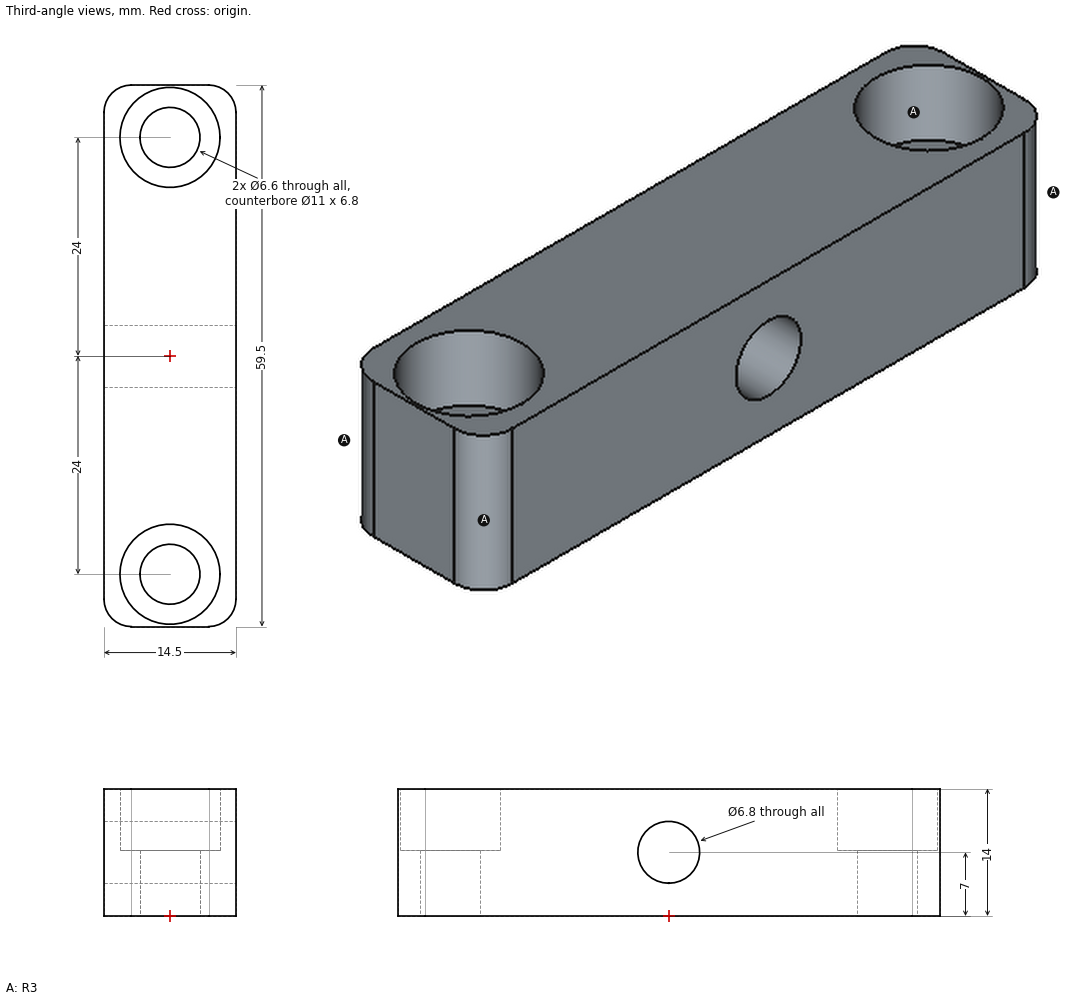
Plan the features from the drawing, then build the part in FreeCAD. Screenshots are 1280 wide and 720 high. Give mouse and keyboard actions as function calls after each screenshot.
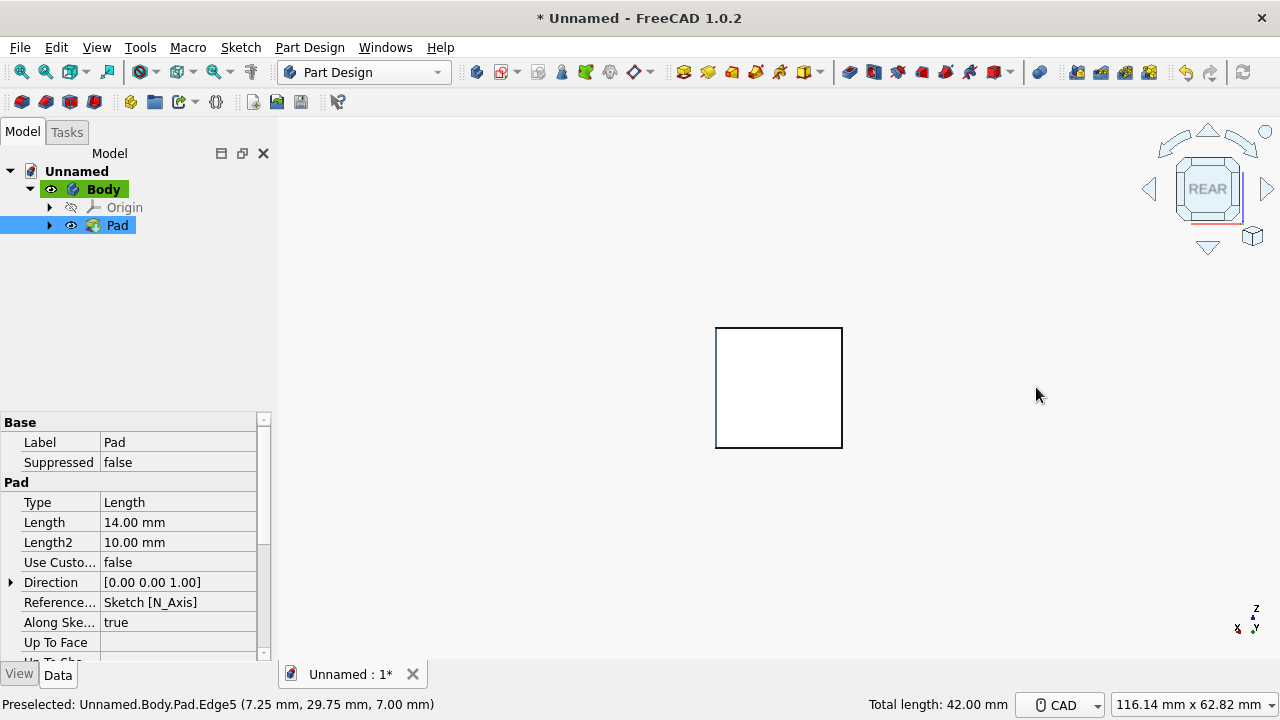
key(v)
key(f)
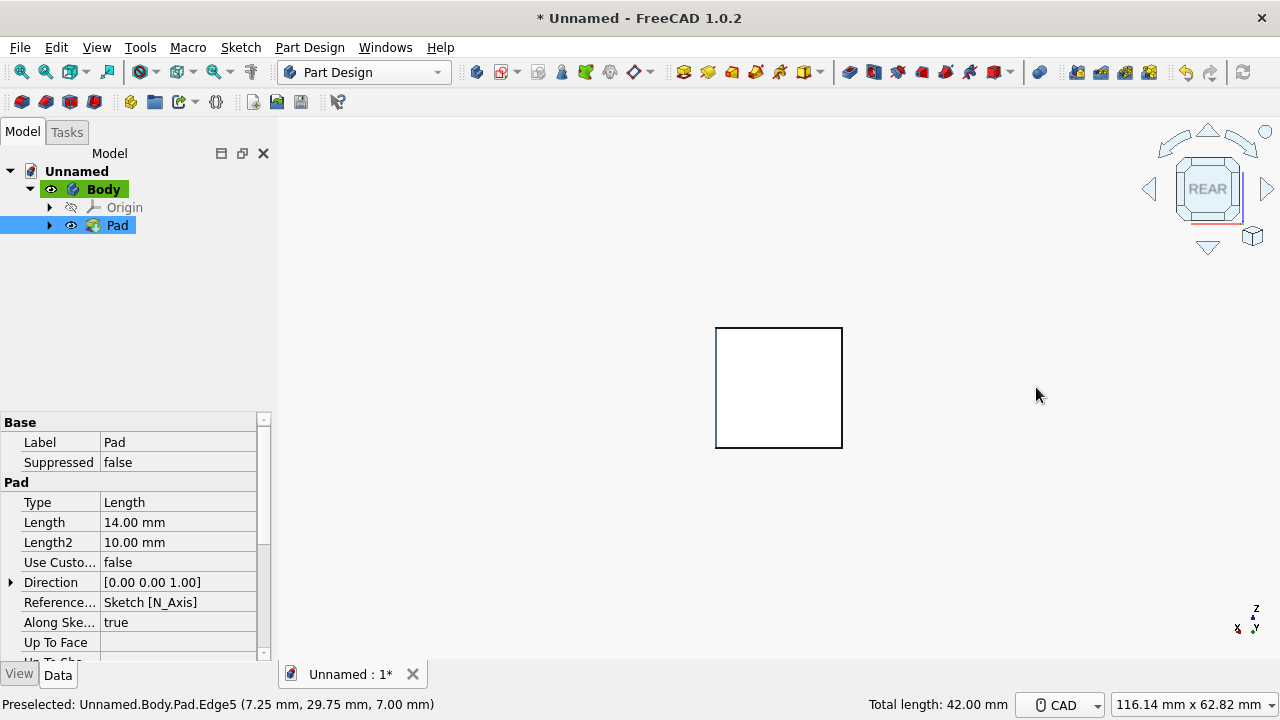
click(842, 387, ctrl)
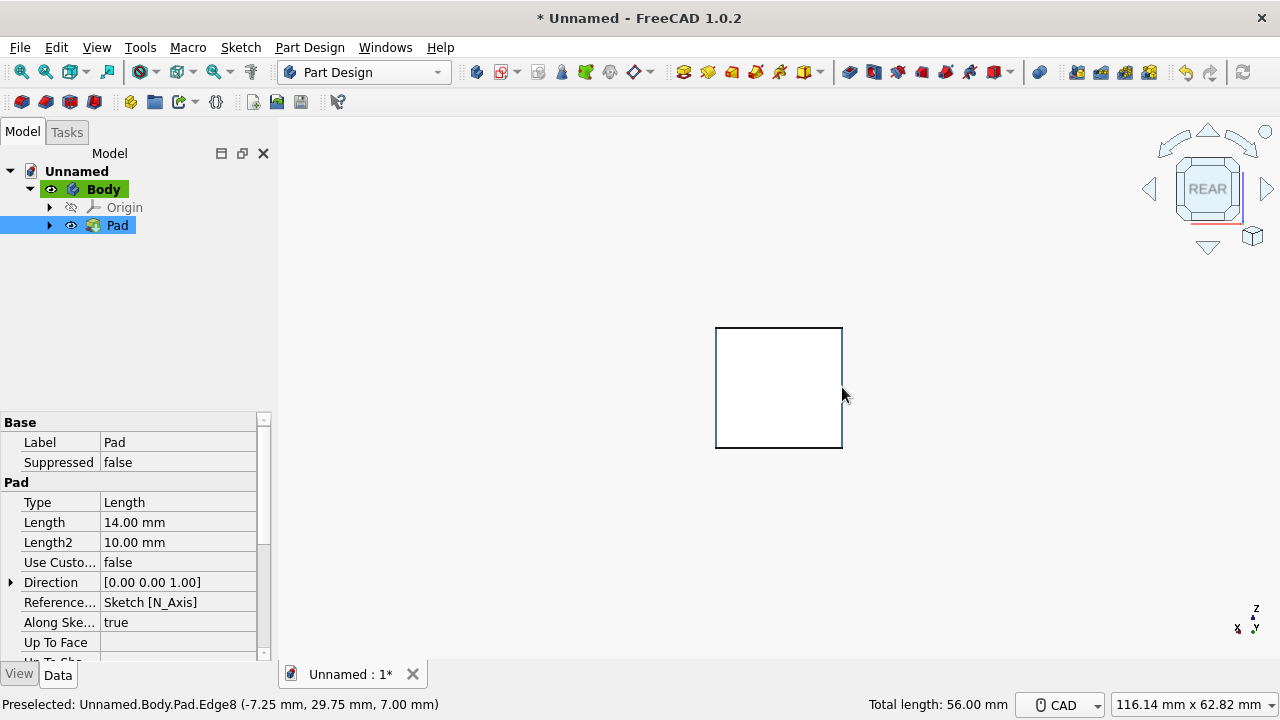
click(22, 102)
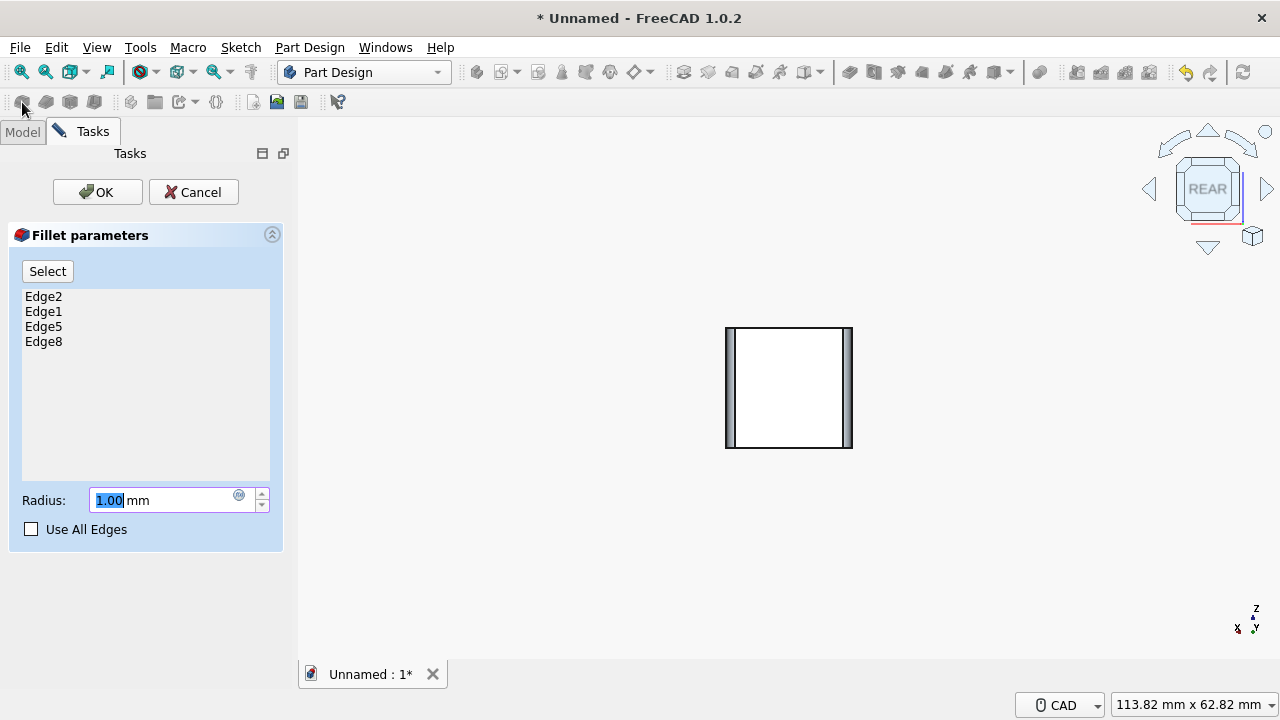
text(3)
key(Tab)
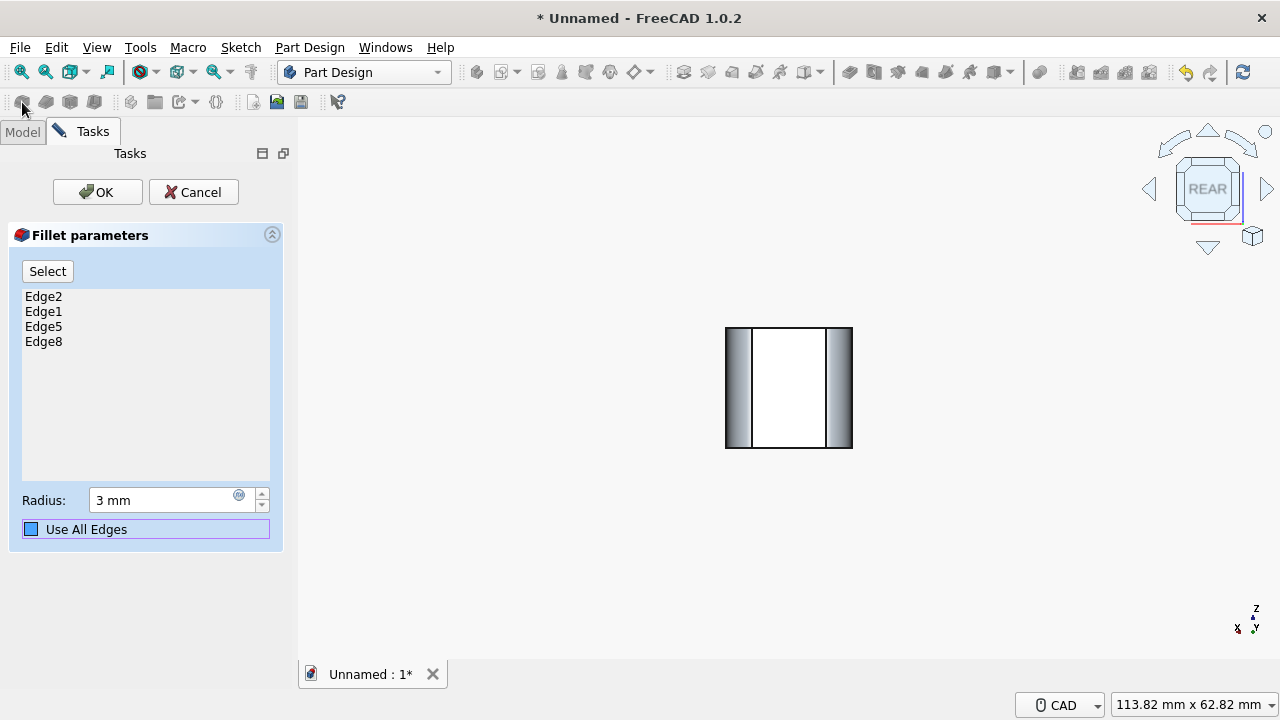
click(98, 192)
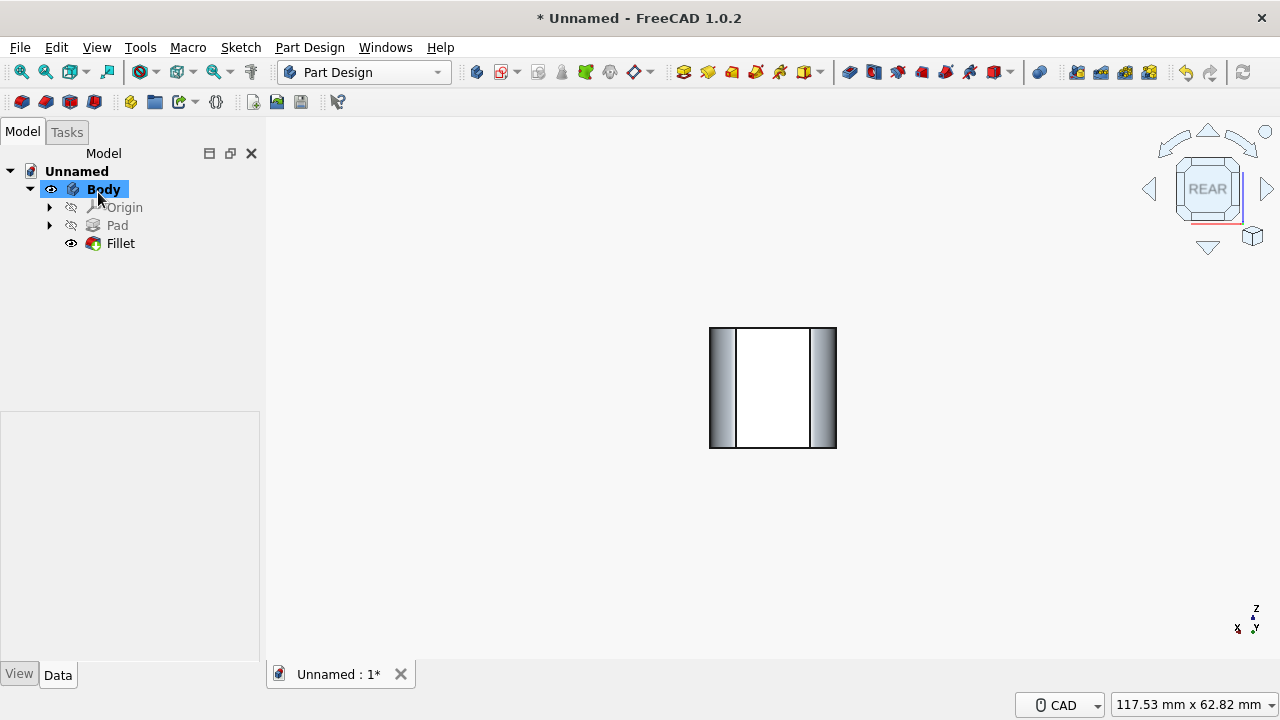
click(22, 72)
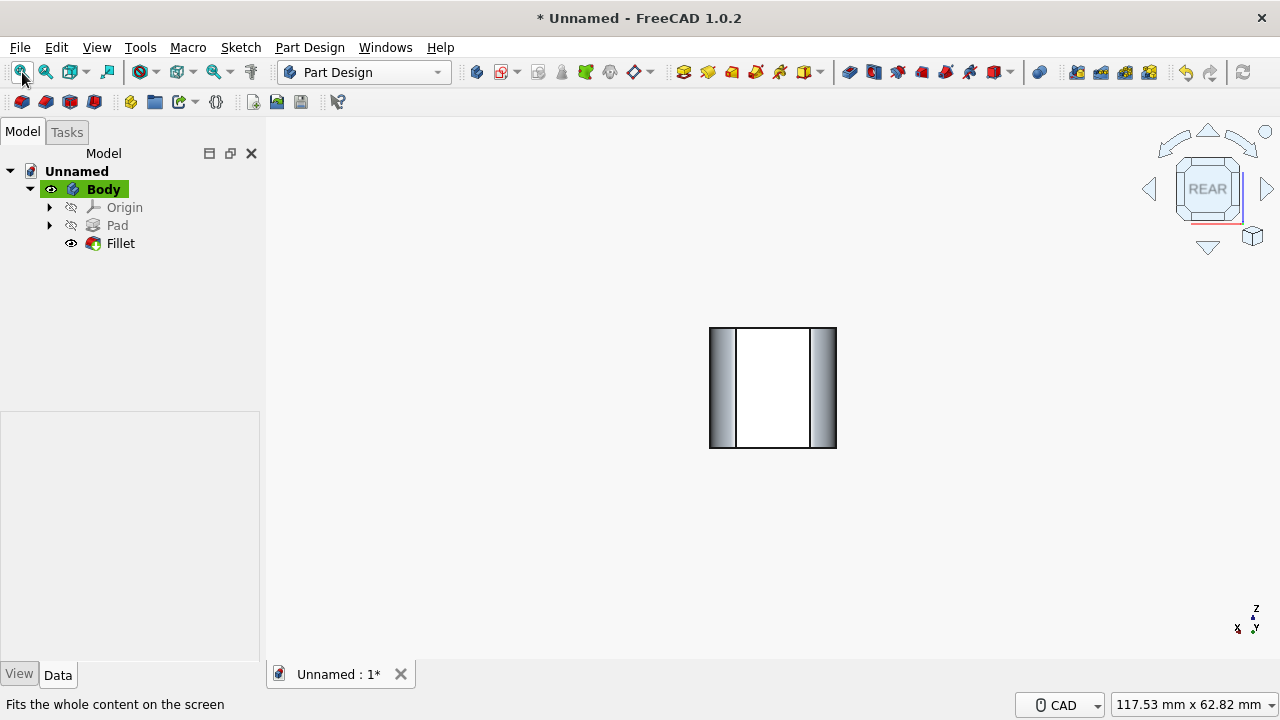
key(0)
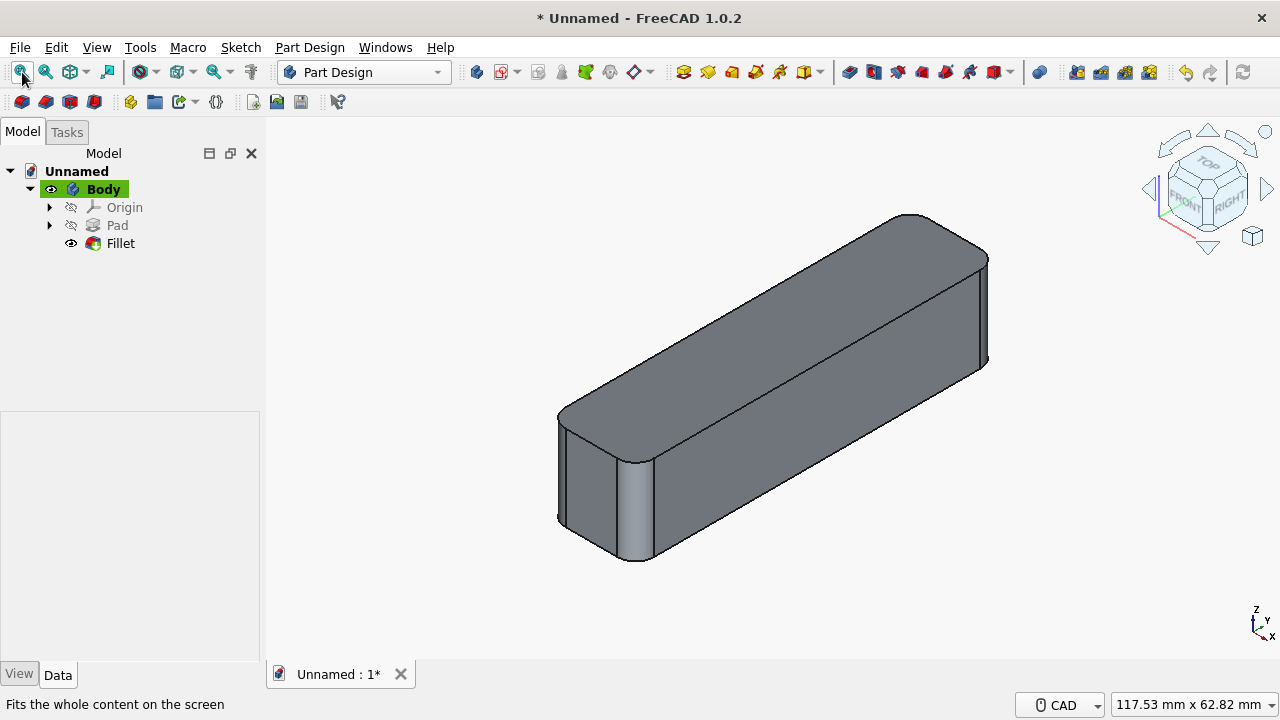
click(877, 278)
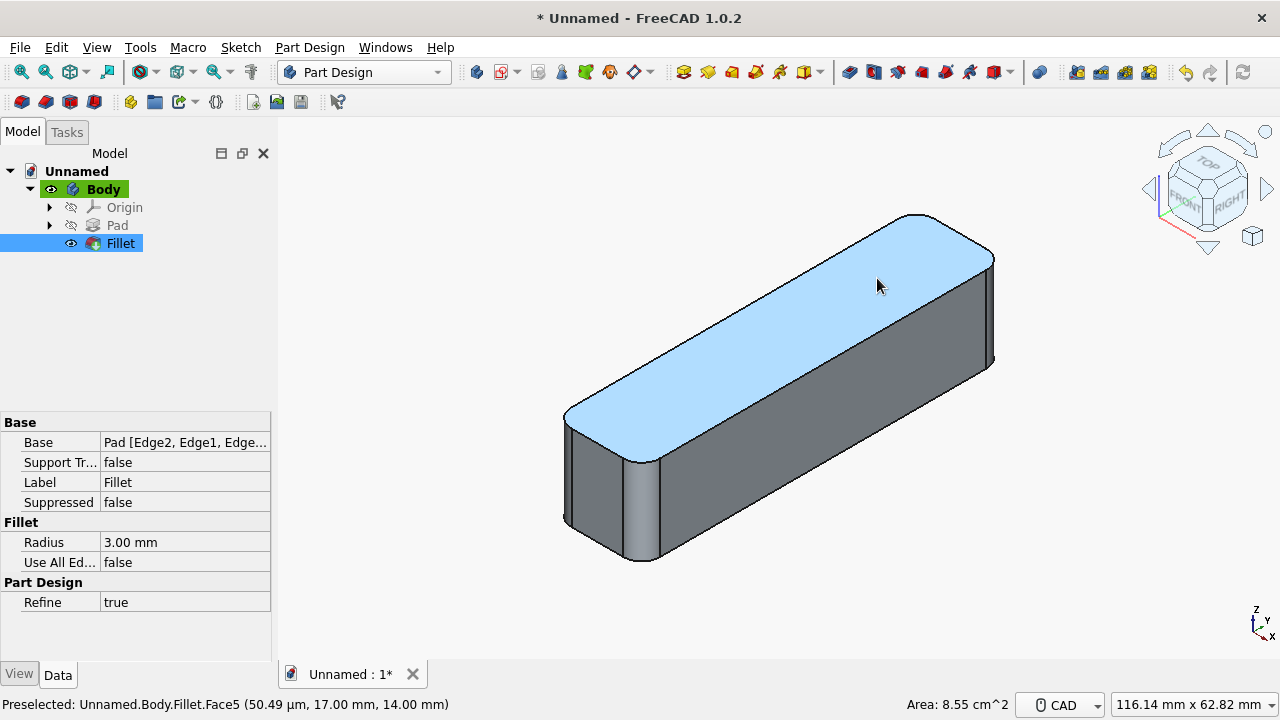
click(502, 72)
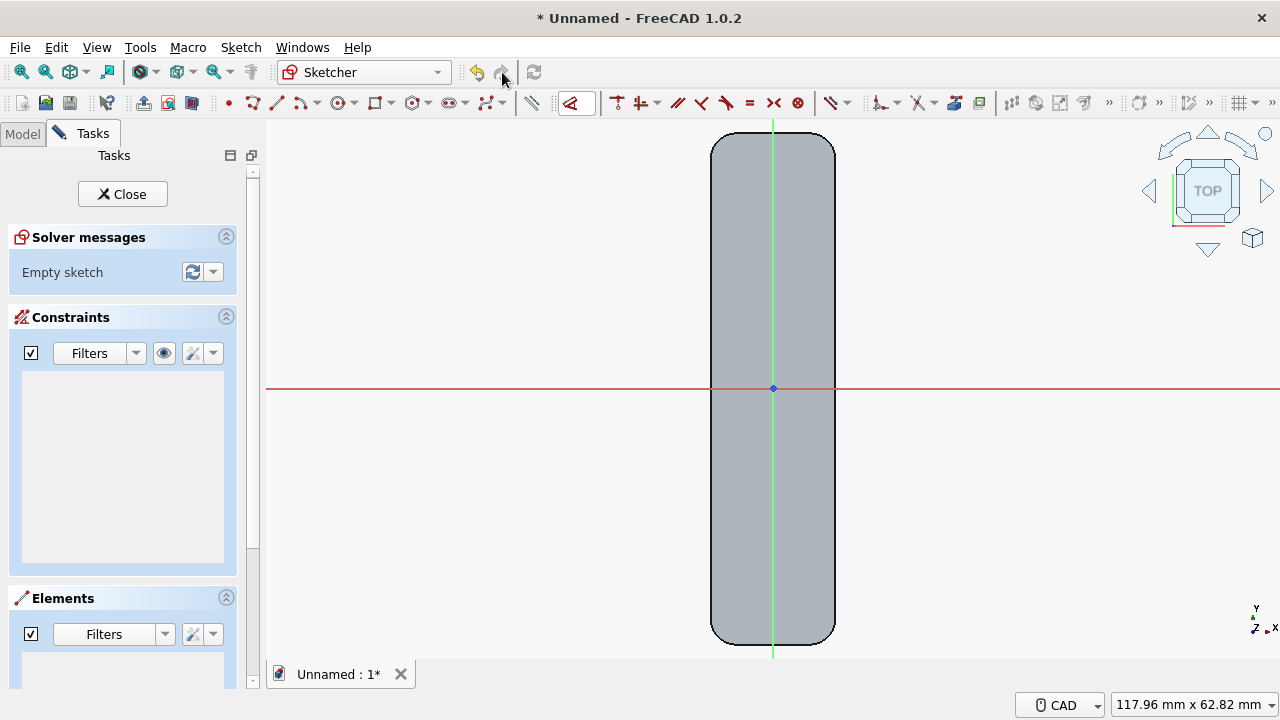
scroll(565, 389, down, 2)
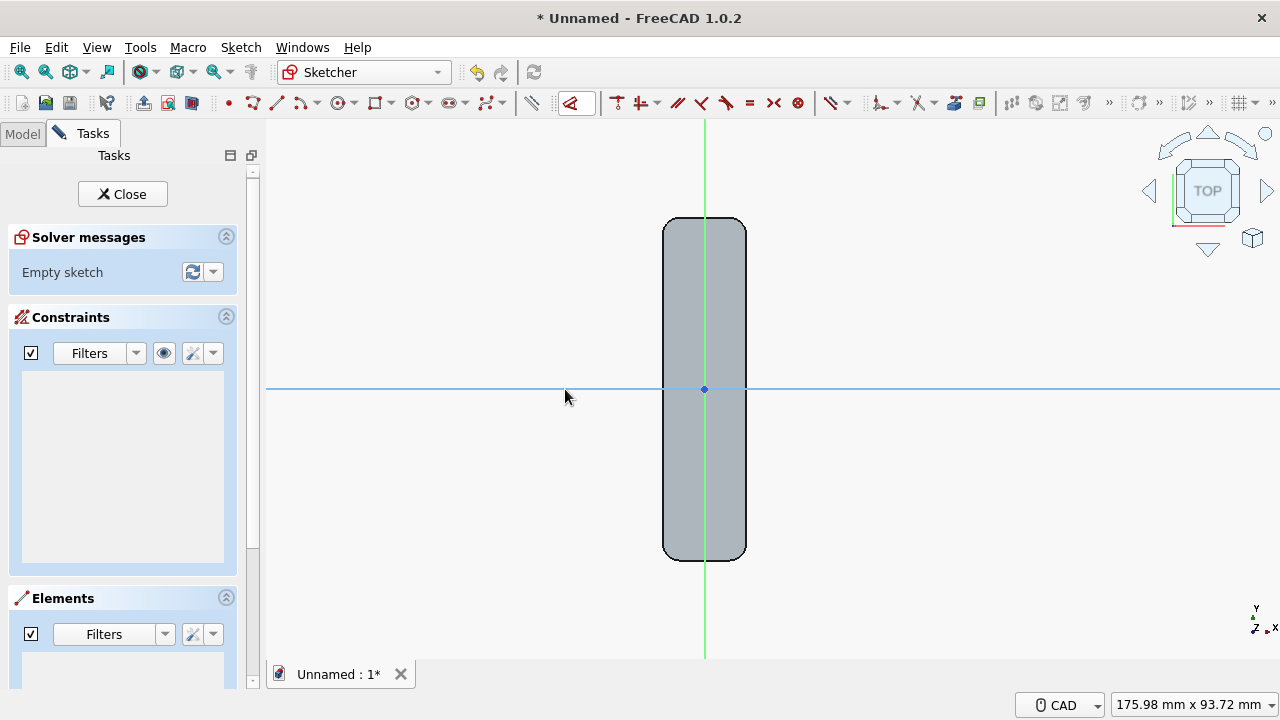
key(g)
key(c)